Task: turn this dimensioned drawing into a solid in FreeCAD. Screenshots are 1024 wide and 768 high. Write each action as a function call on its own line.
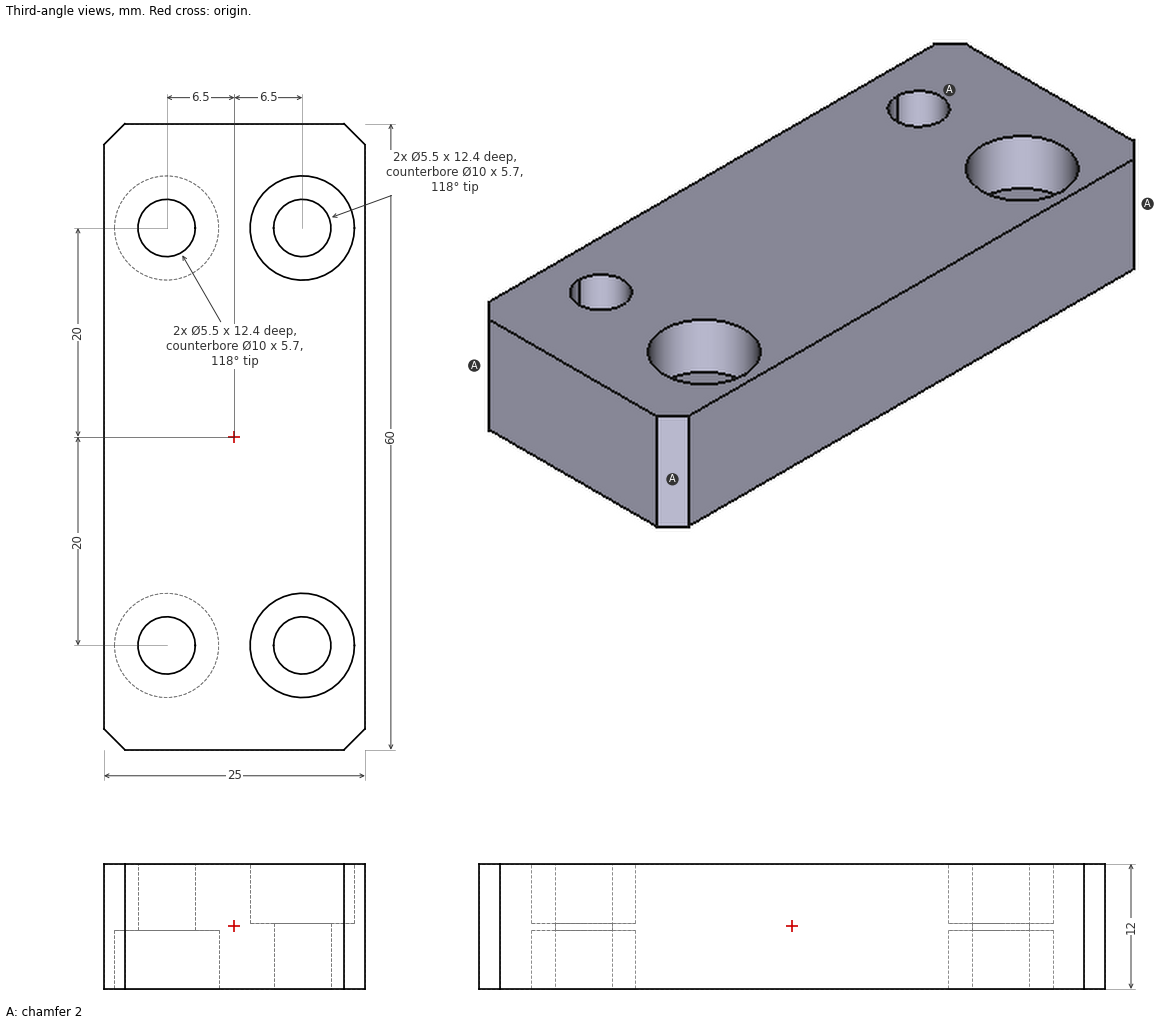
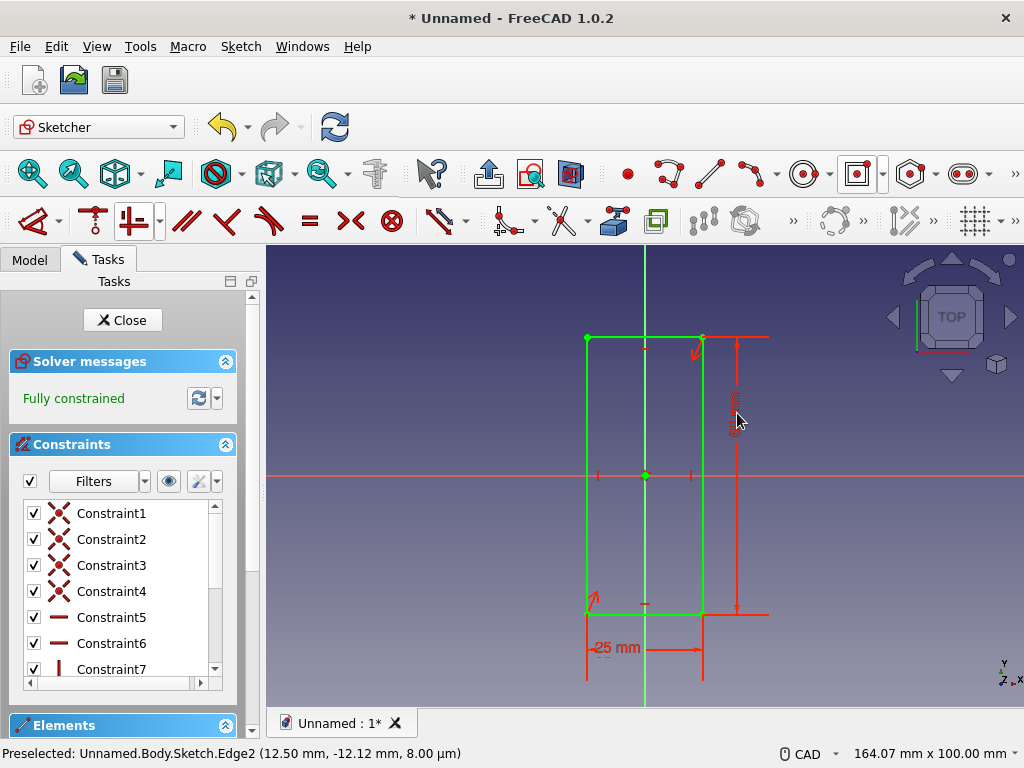
click(123, 320)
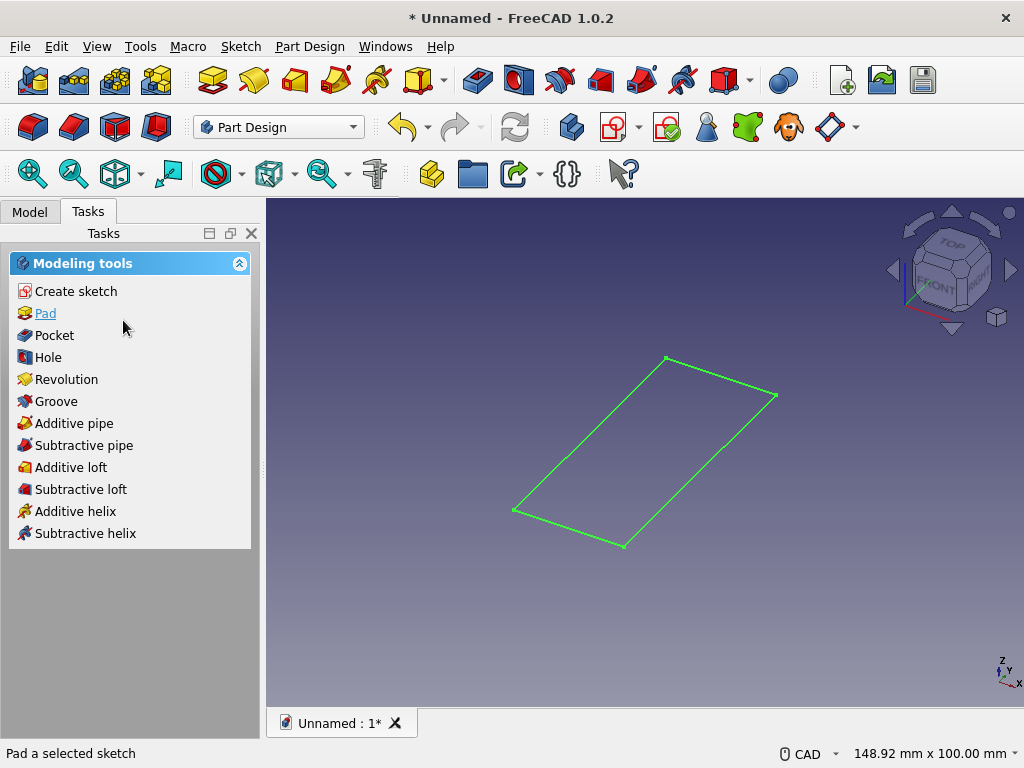
click(213, 80)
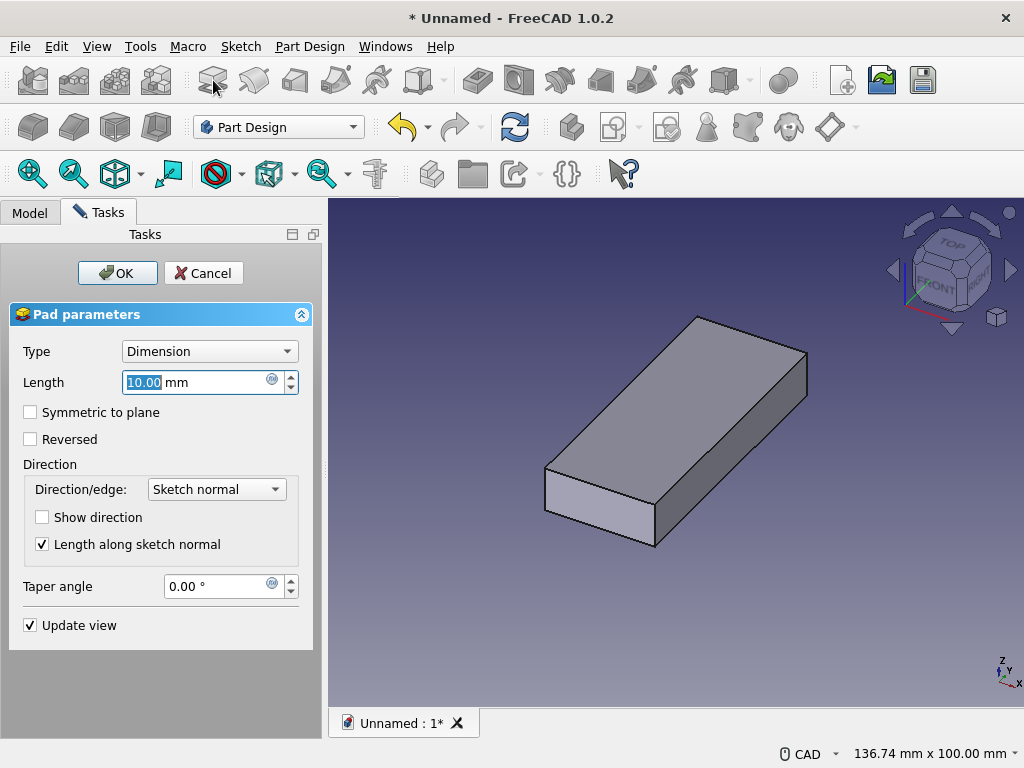
text(12)
key(Tab)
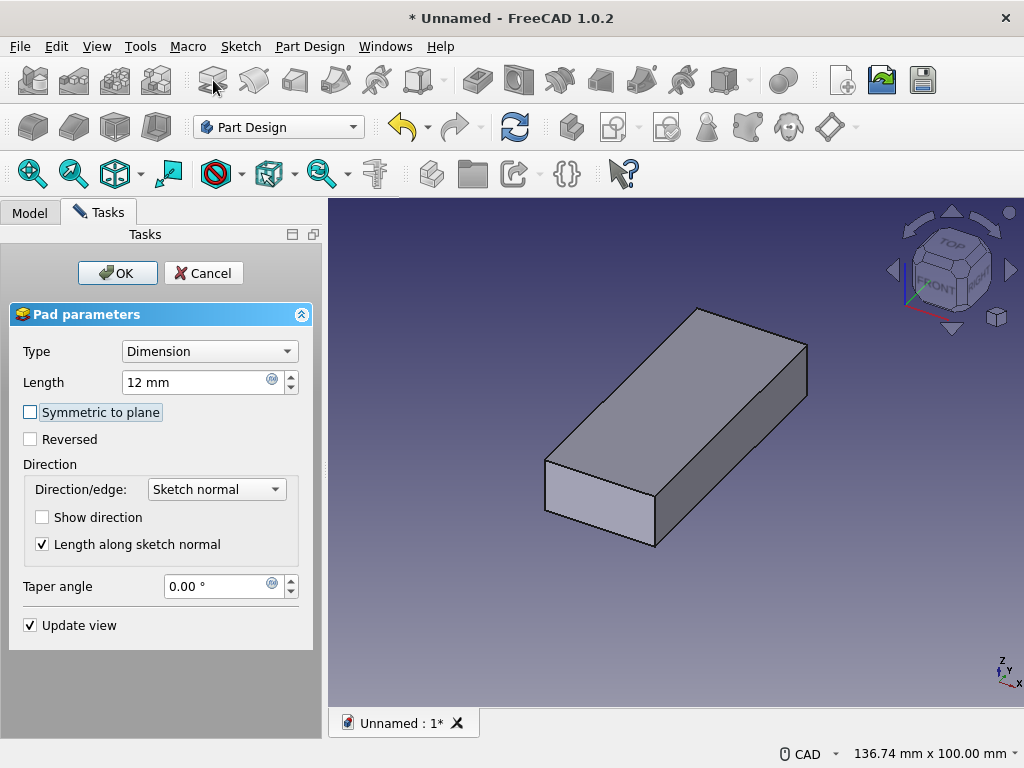
click(31, 412)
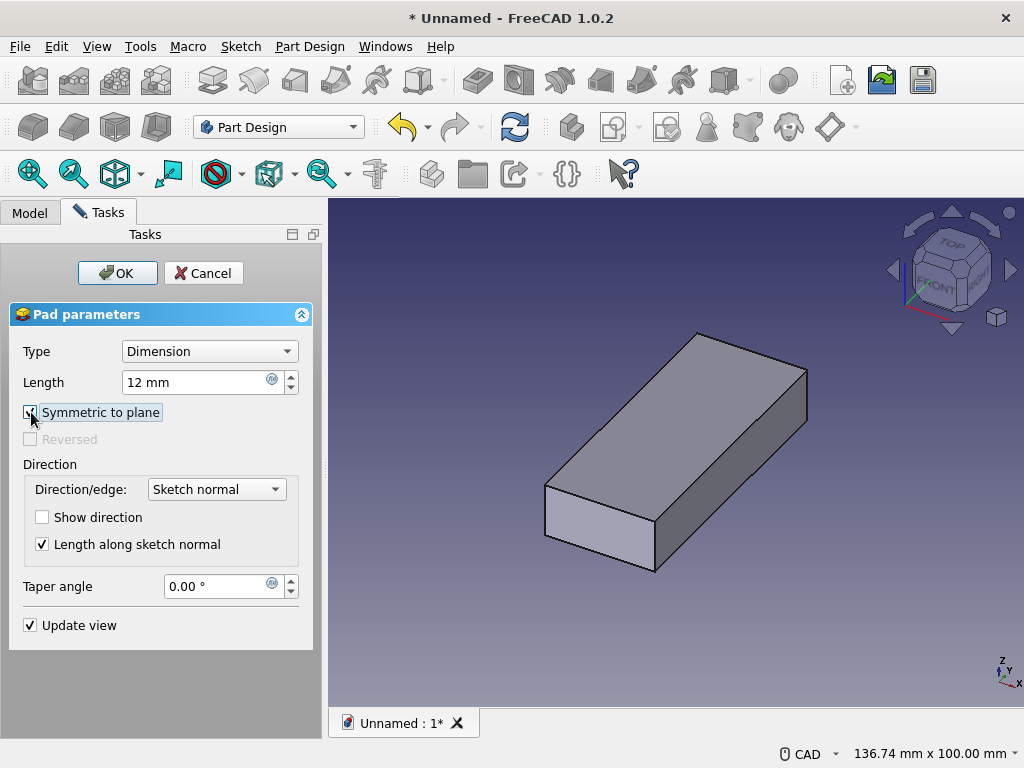
click(118, 273)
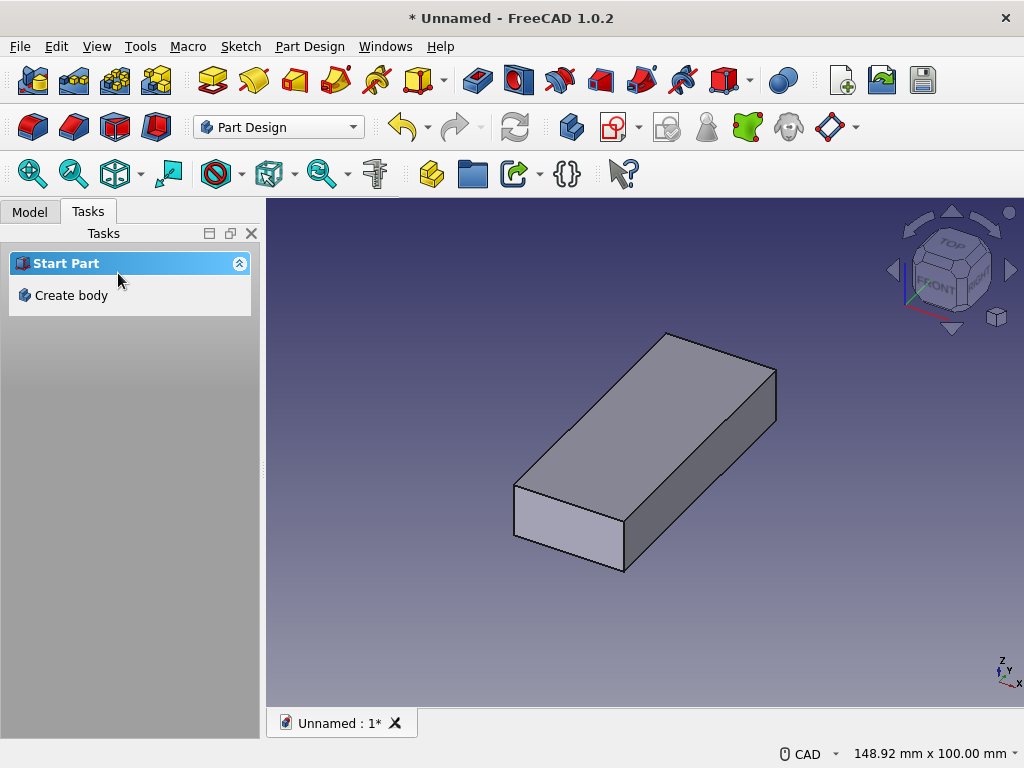
click(624, 546)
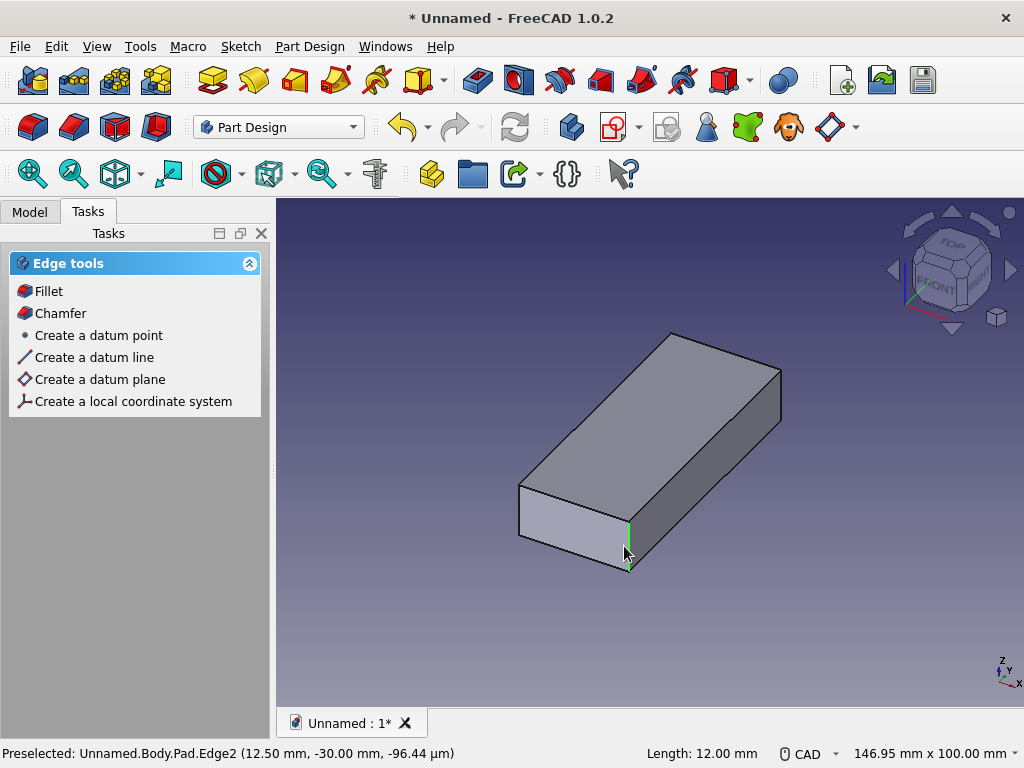
key(0)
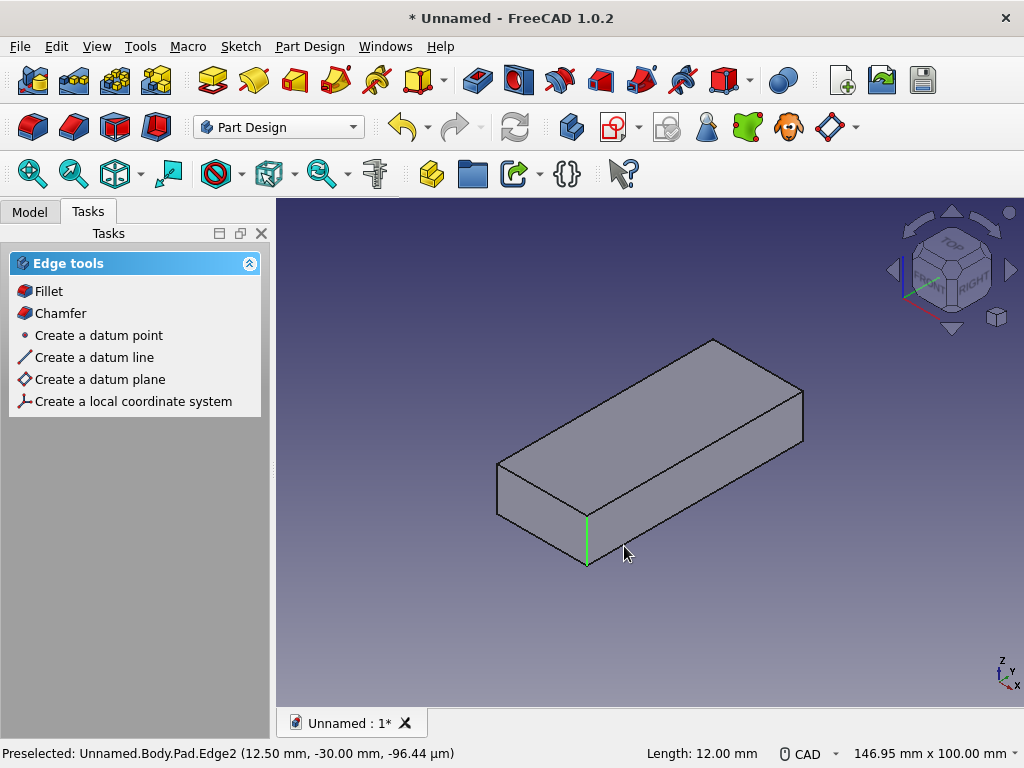
click(33, 174)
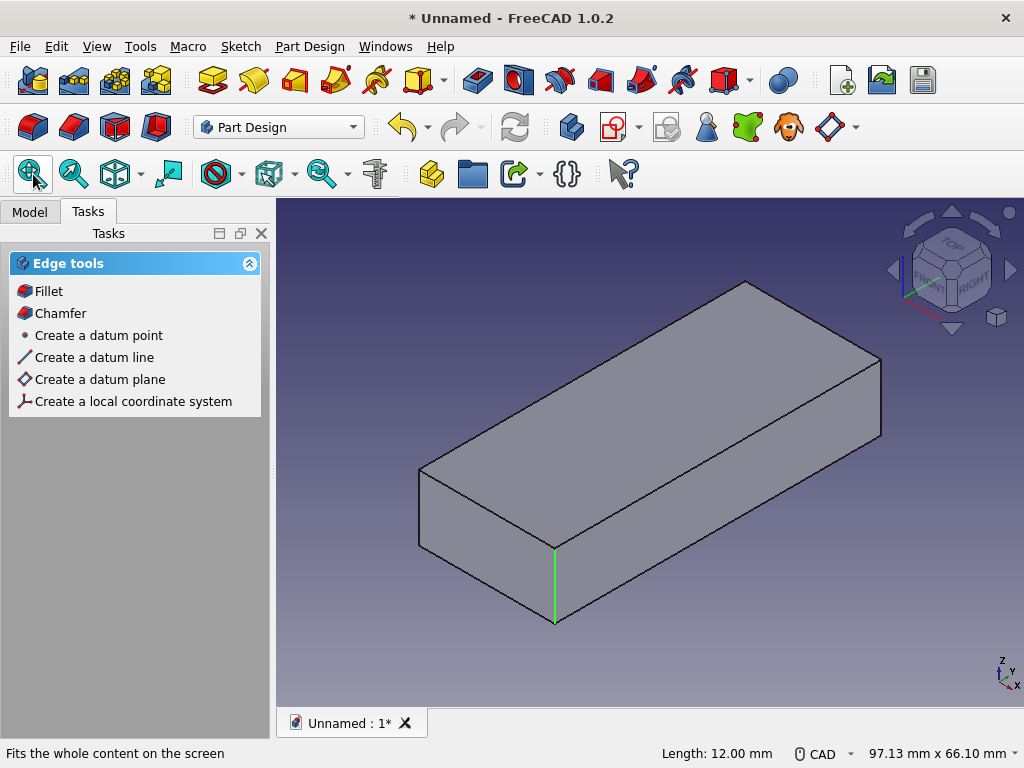
key(2)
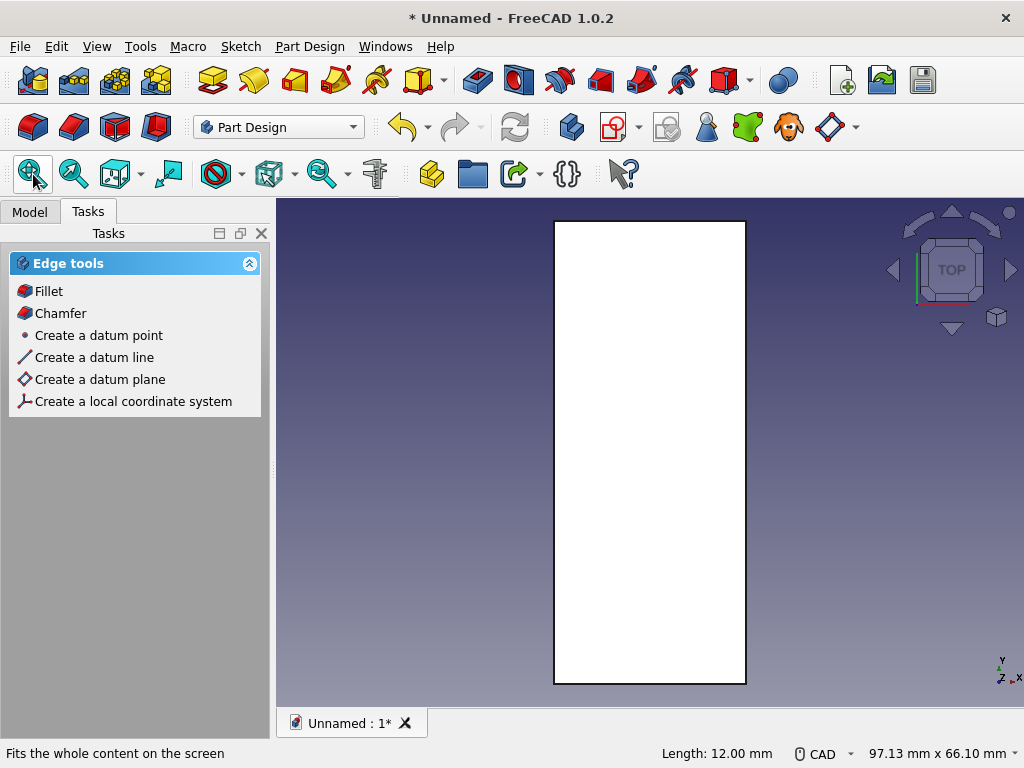
key(1)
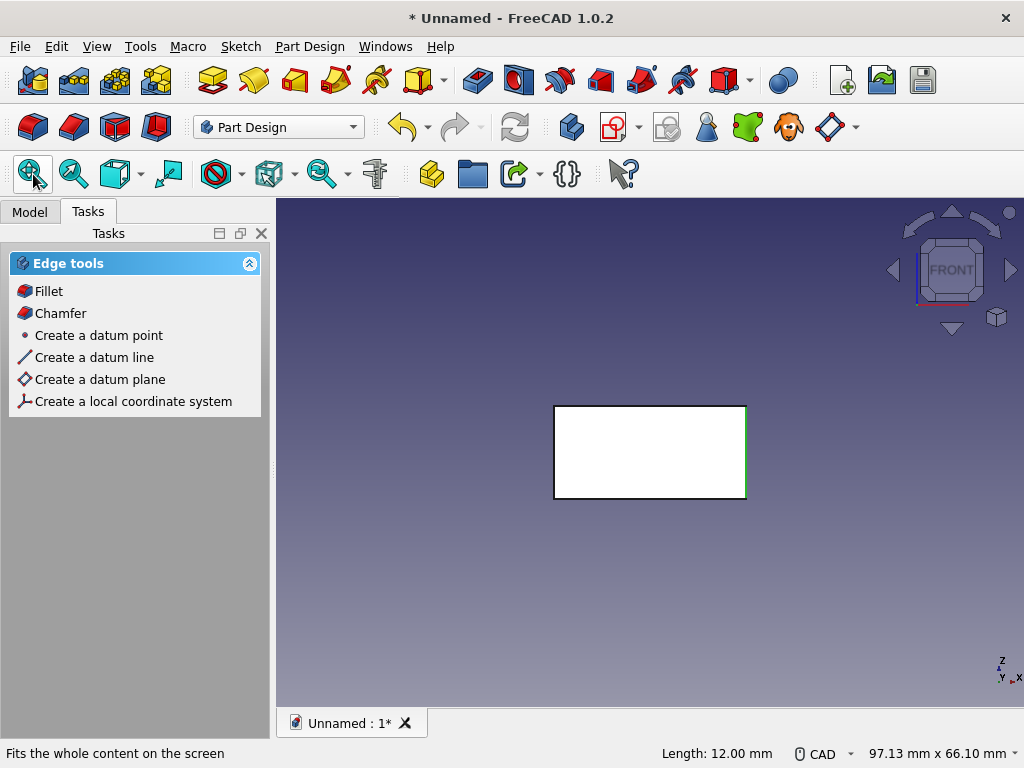
click(33, 174)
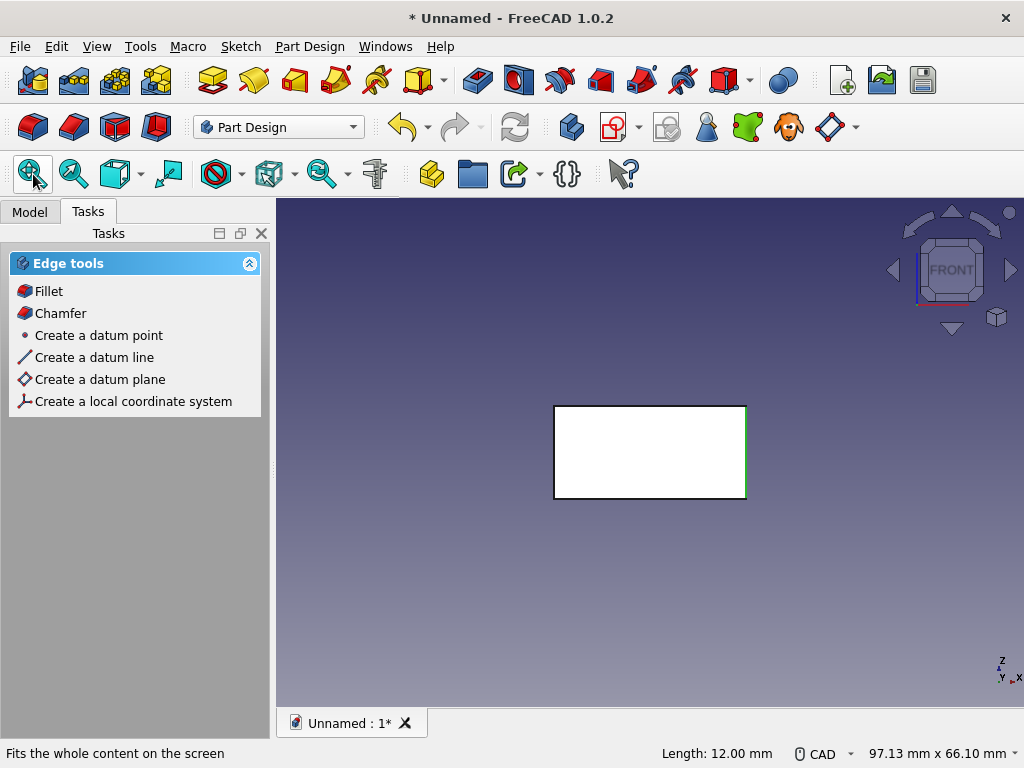
click(554, 452, ctrl)